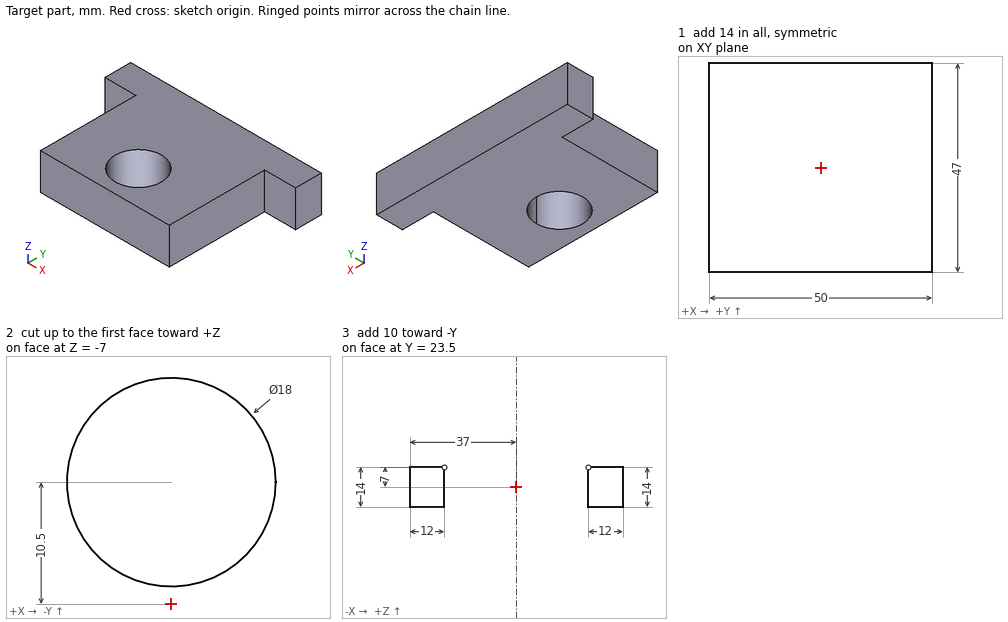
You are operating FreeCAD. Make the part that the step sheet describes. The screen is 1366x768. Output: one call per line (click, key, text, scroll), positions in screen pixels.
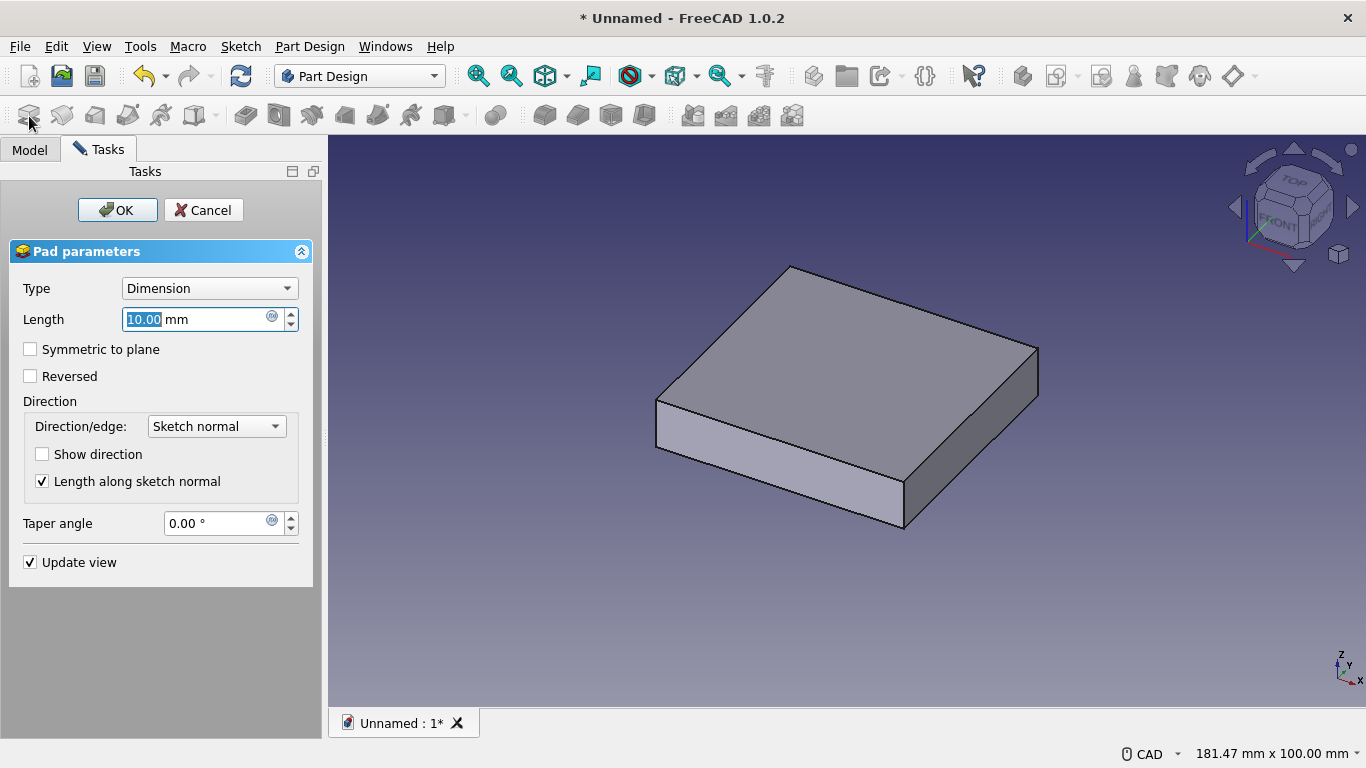
text(14)
key(Tab)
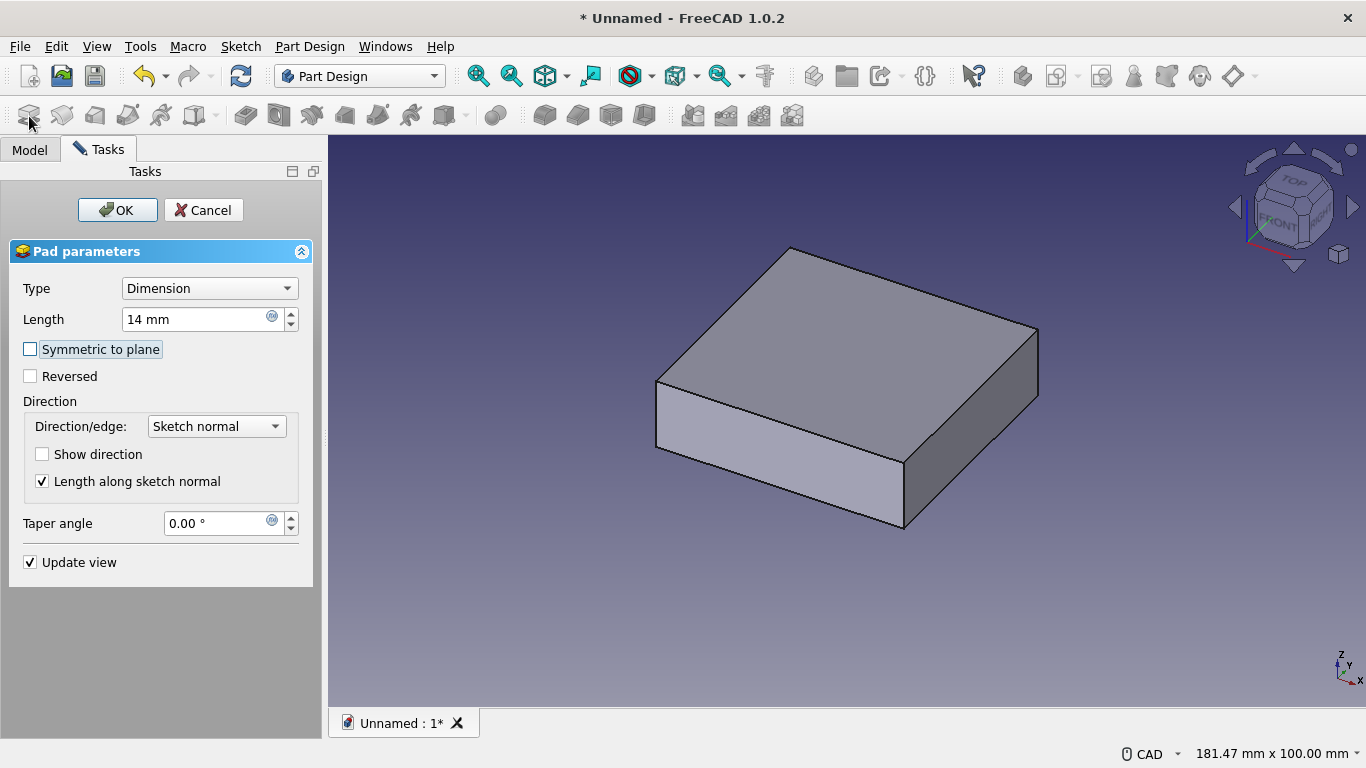
click(31, 349)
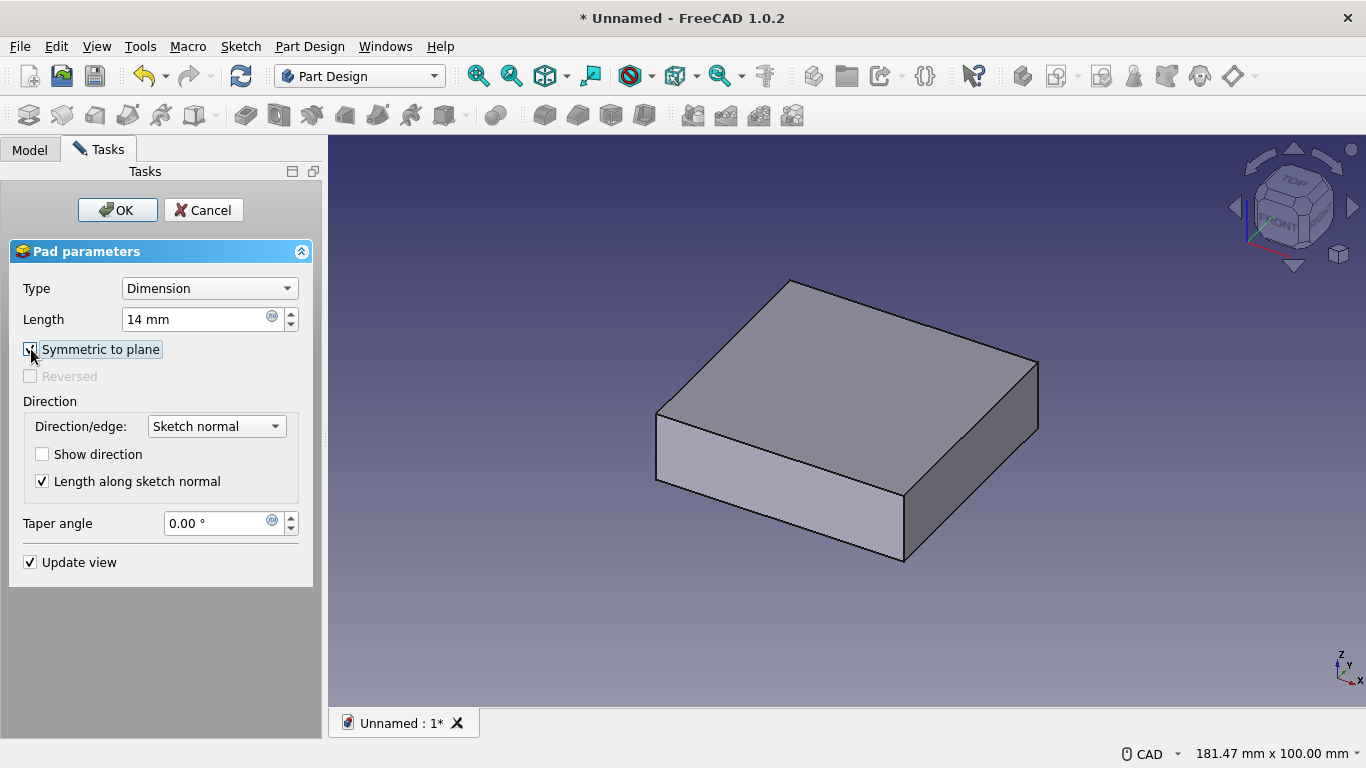
click(118, 210)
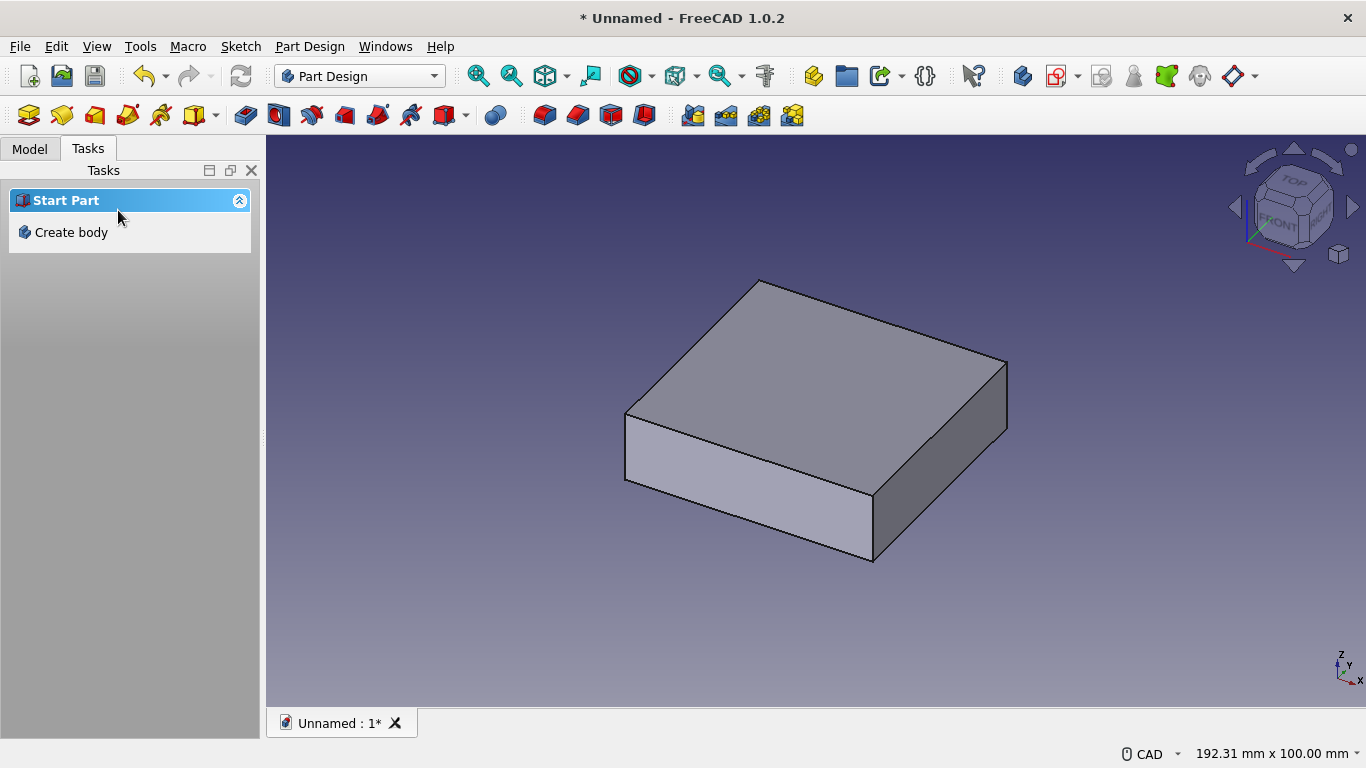
key(5)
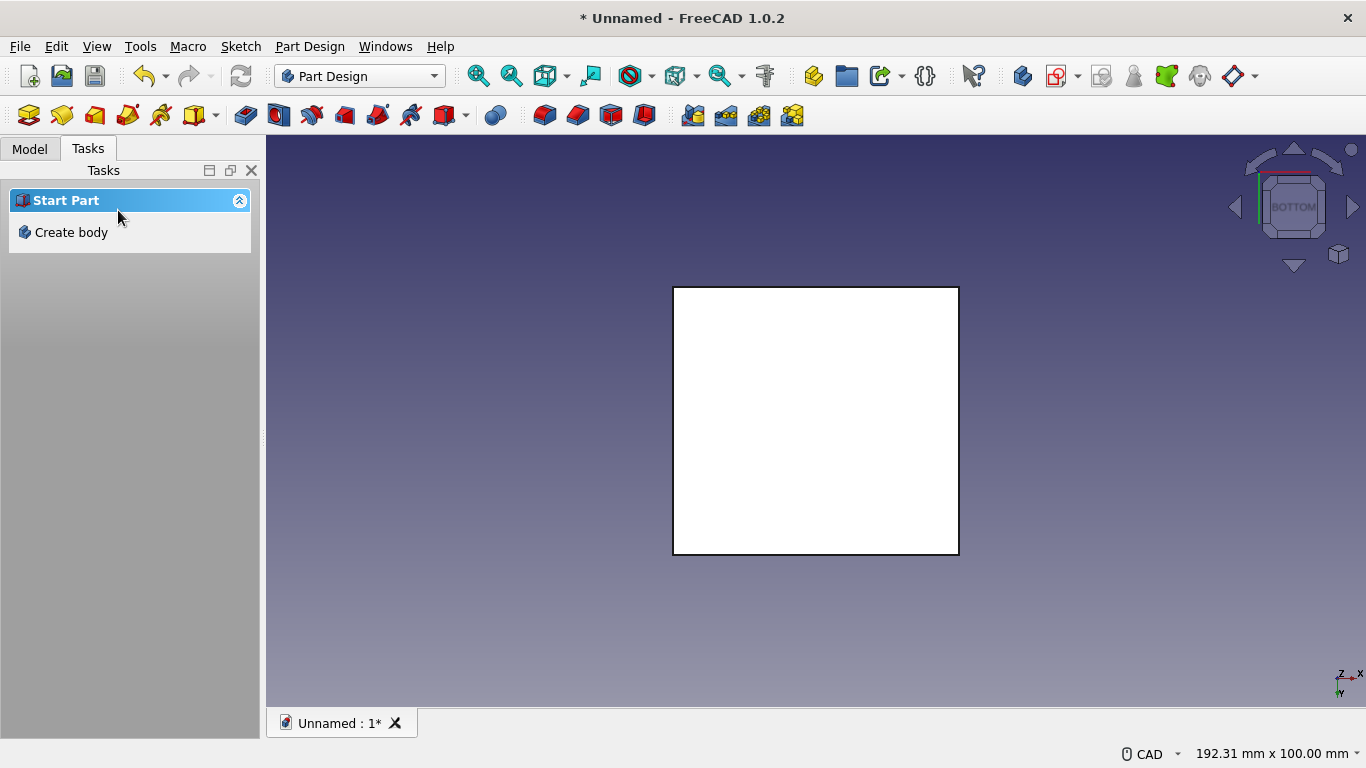
click(816, 420)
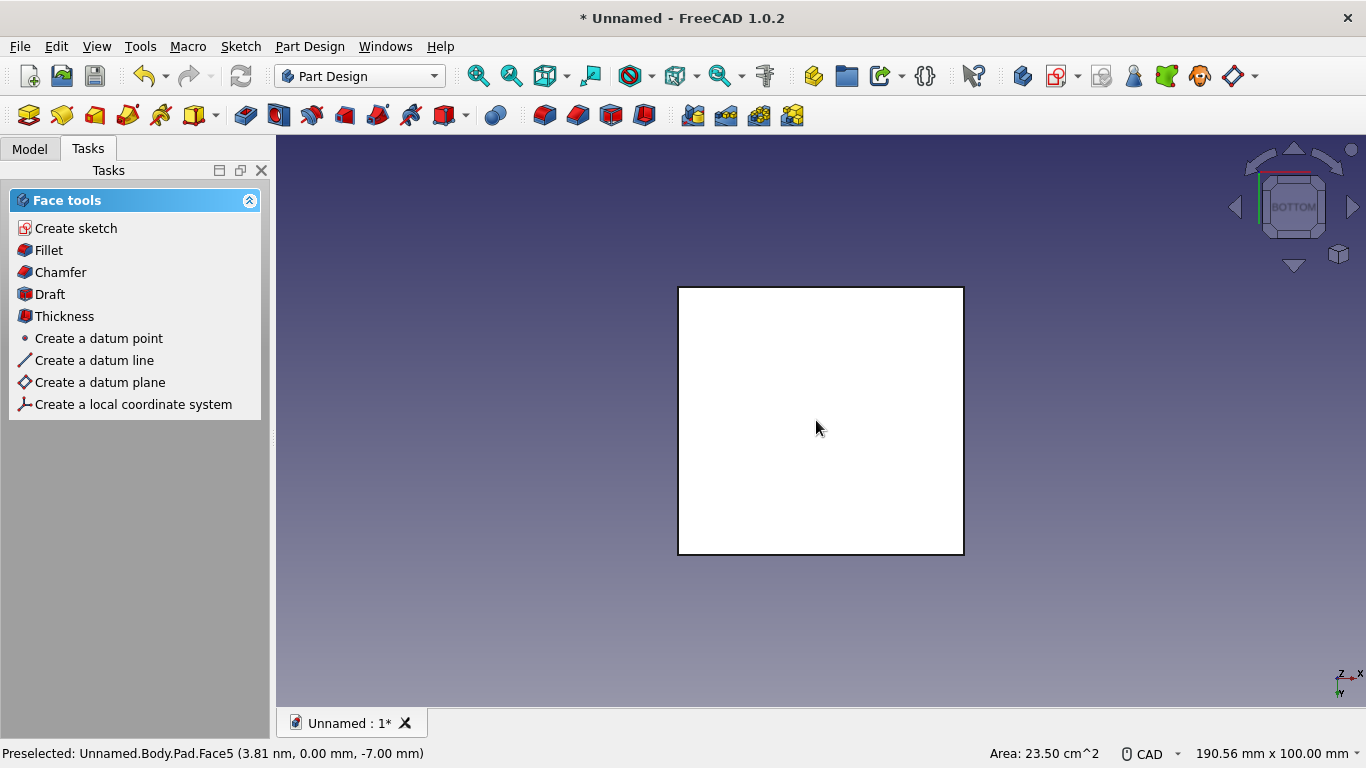
click(1056, 76)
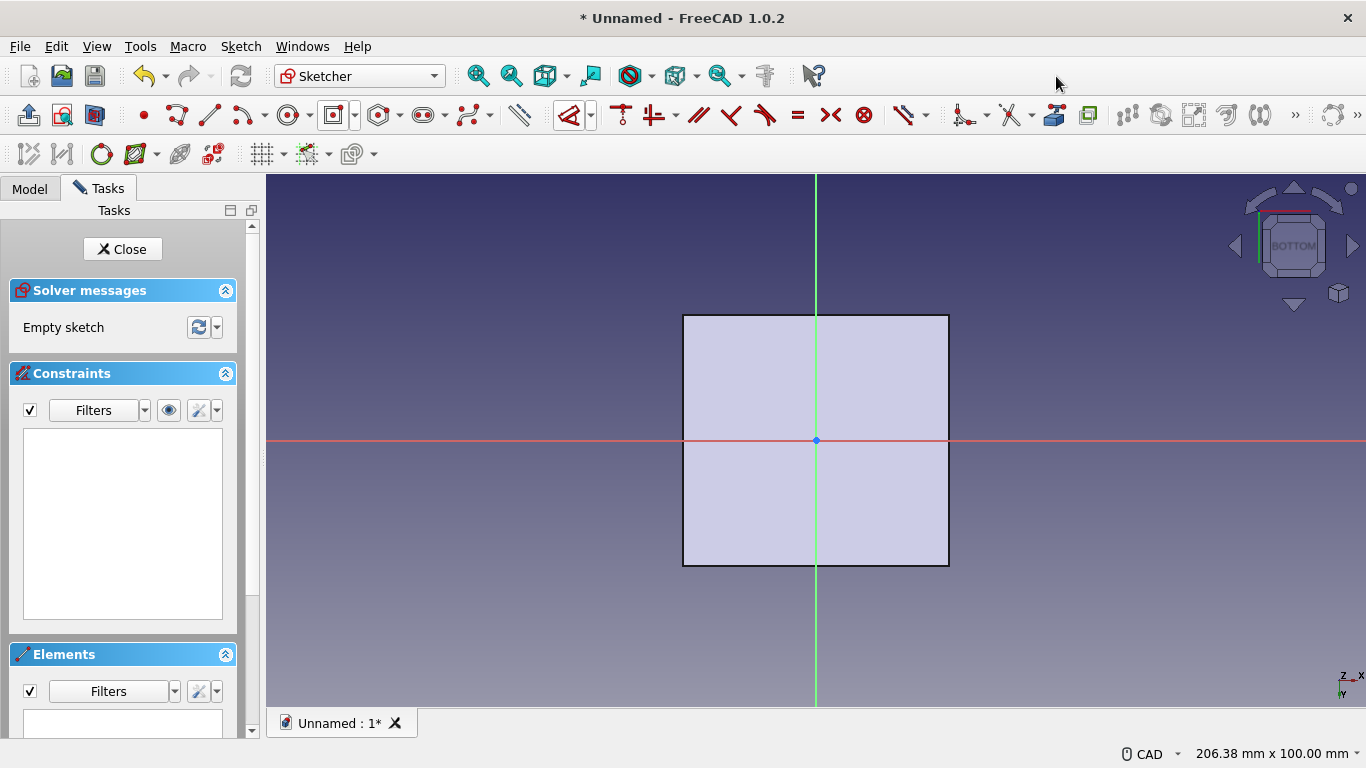
scroll(846, 366, up, 6)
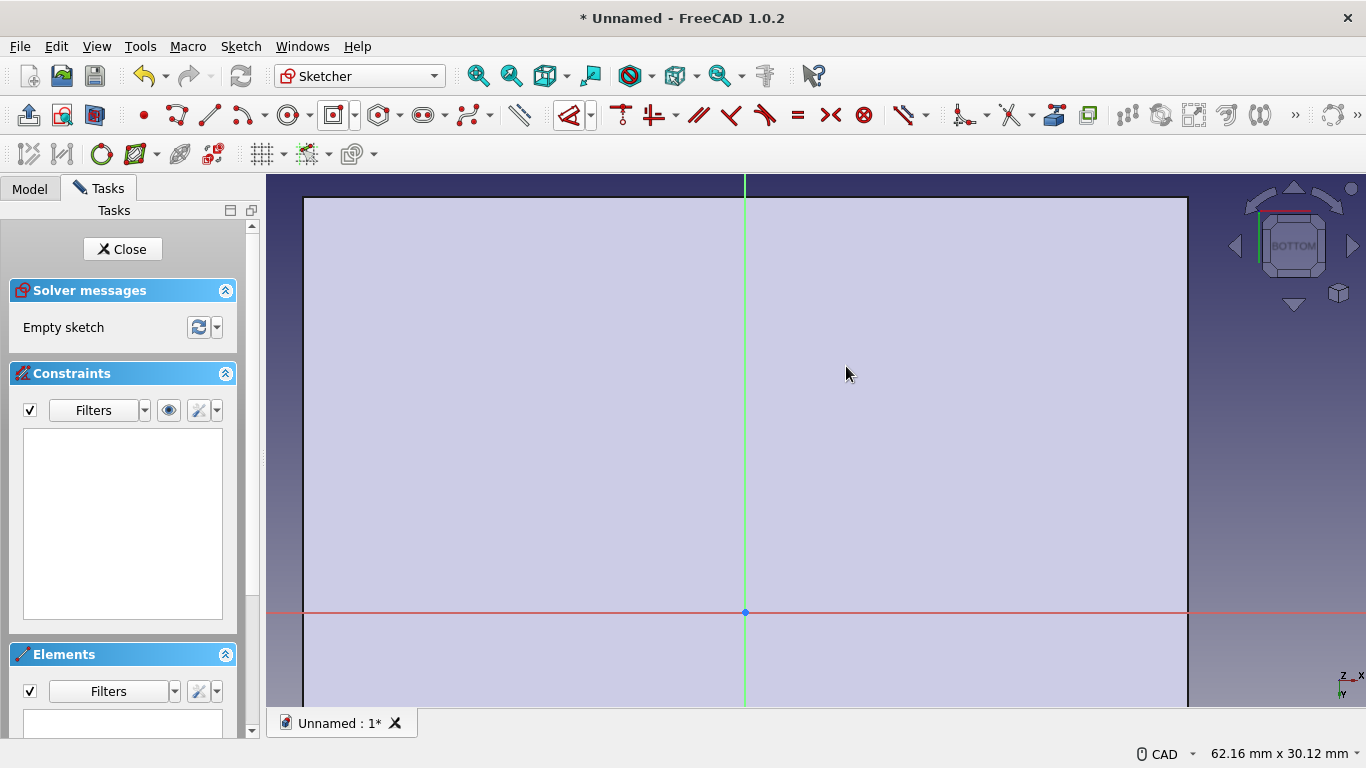
click(288, 116)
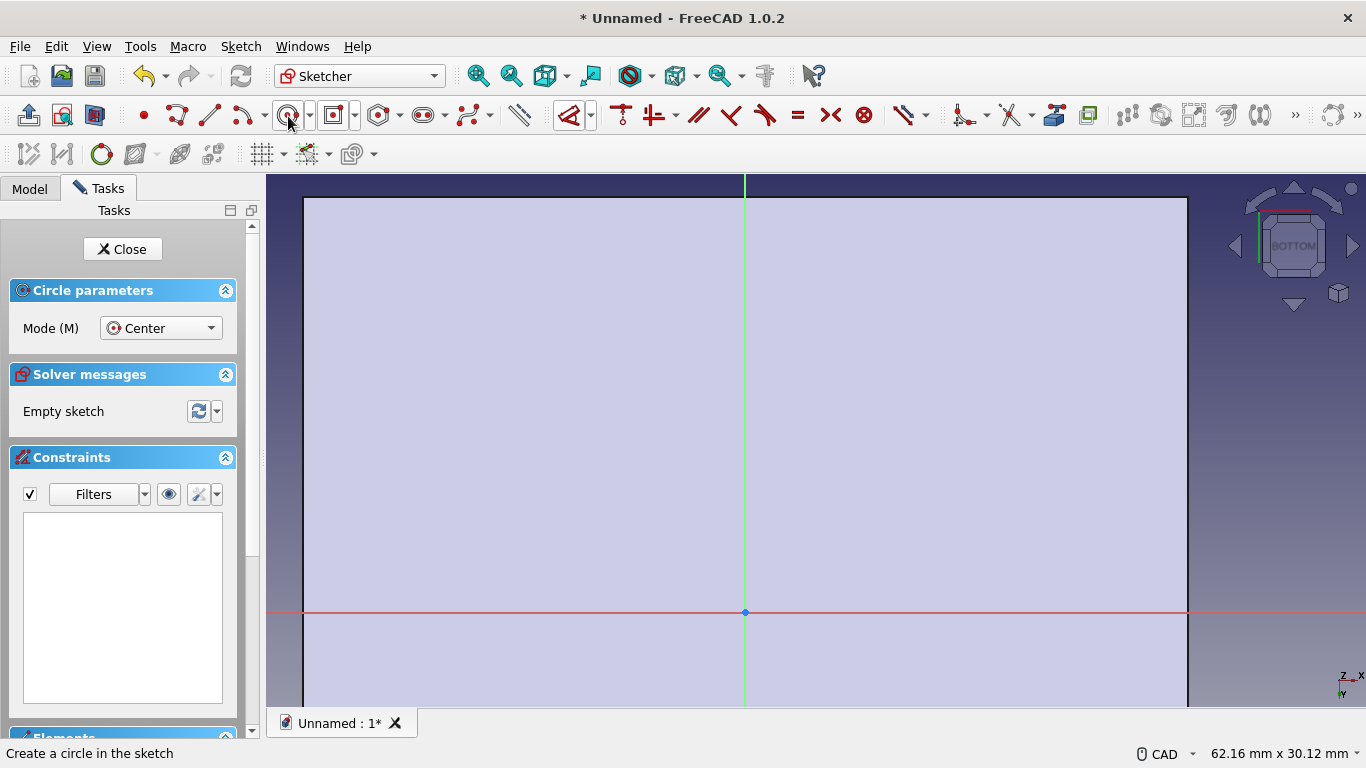
click(745, 427)
move(858, 314)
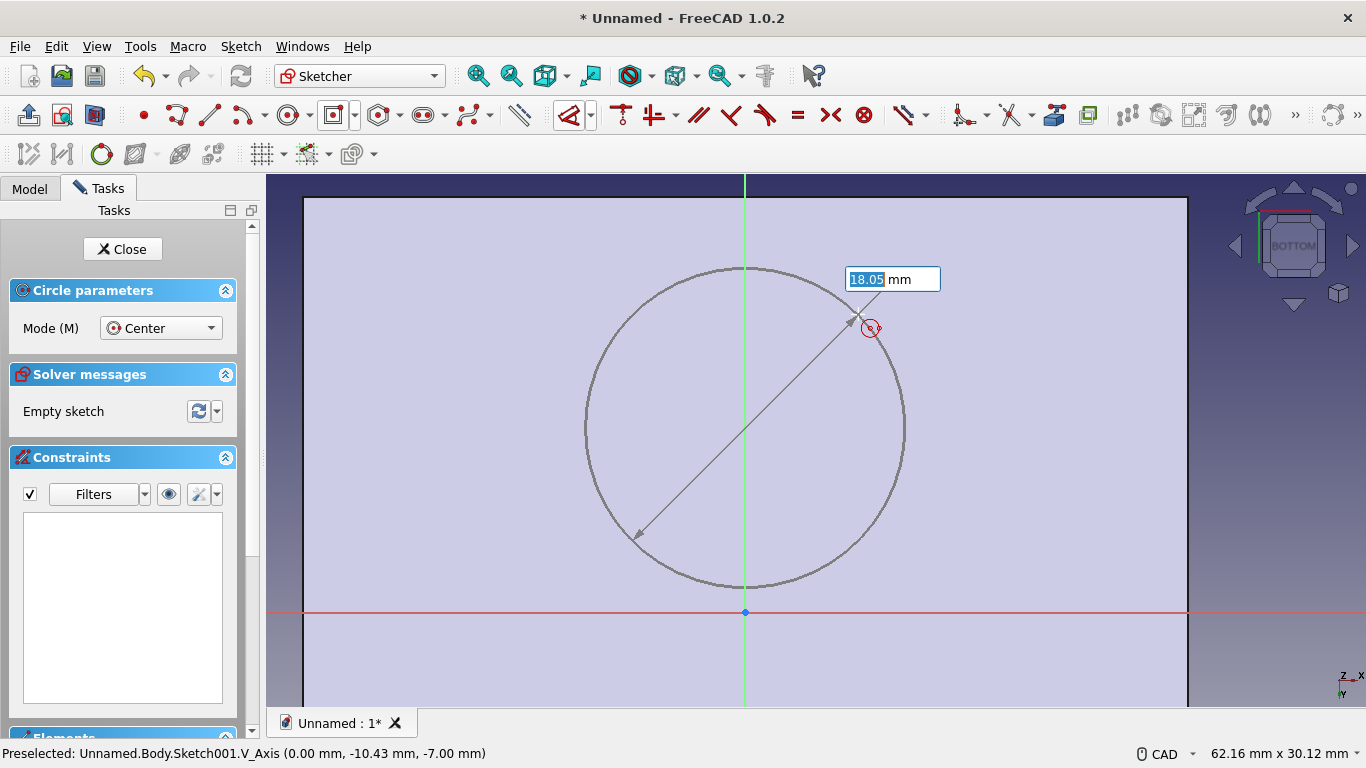
text(18)
key(Return)
key(Escape)